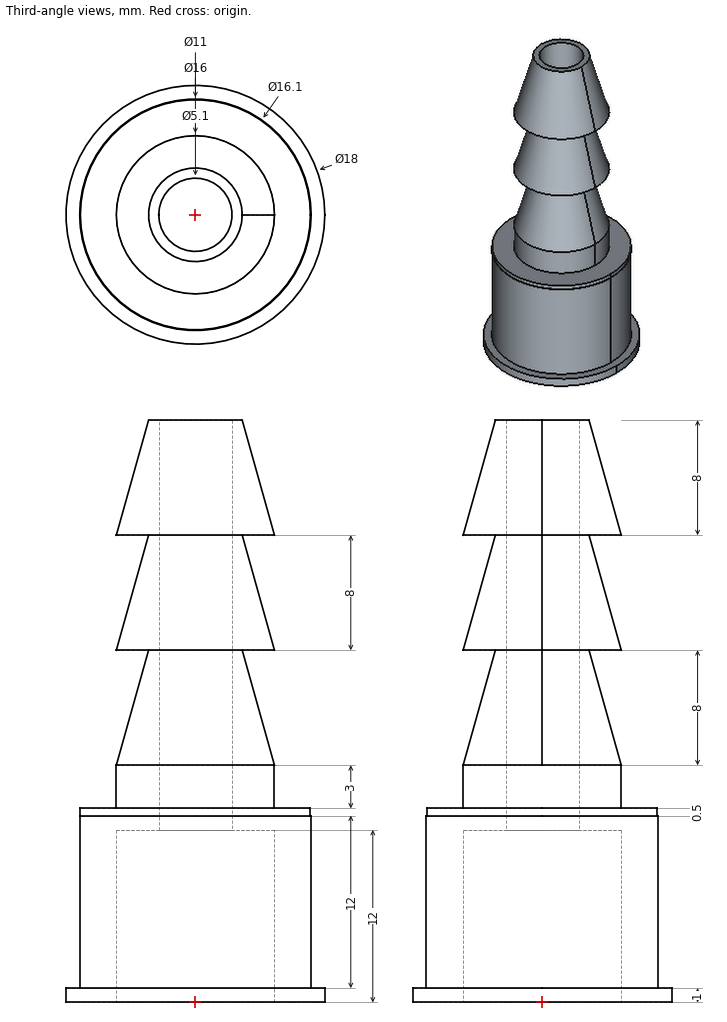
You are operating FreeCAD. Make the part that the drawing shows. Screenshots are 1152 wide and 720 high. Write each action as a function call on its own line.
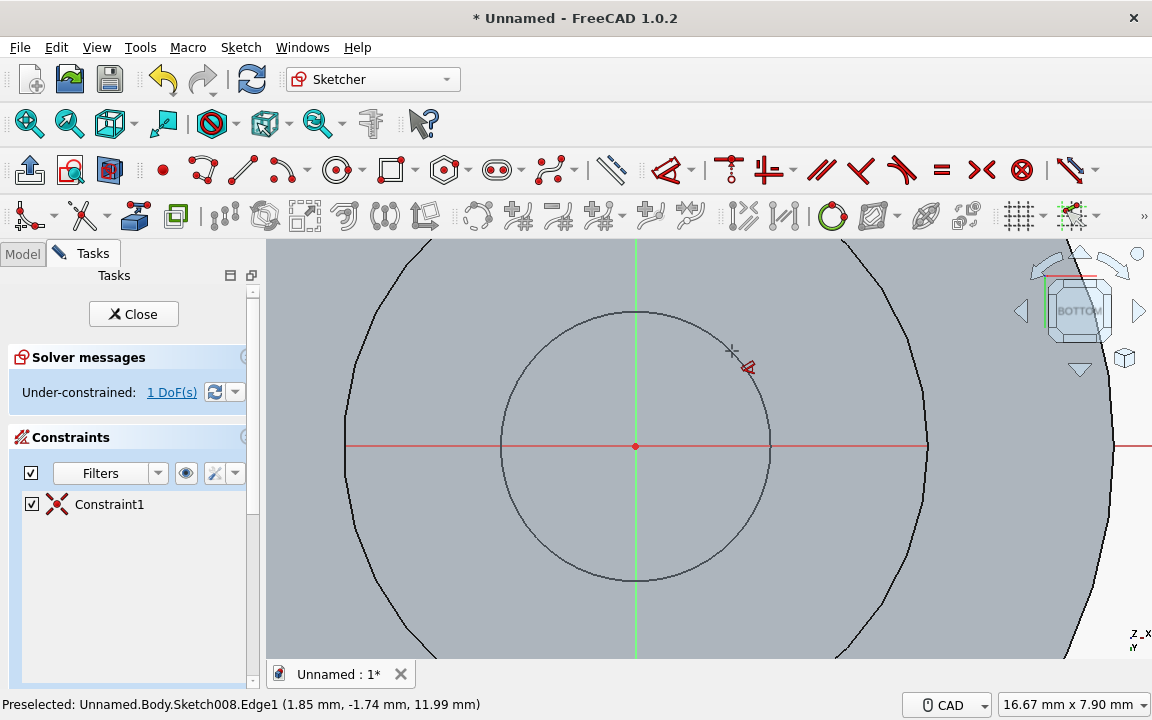
click(731, 351)
click(754, 328)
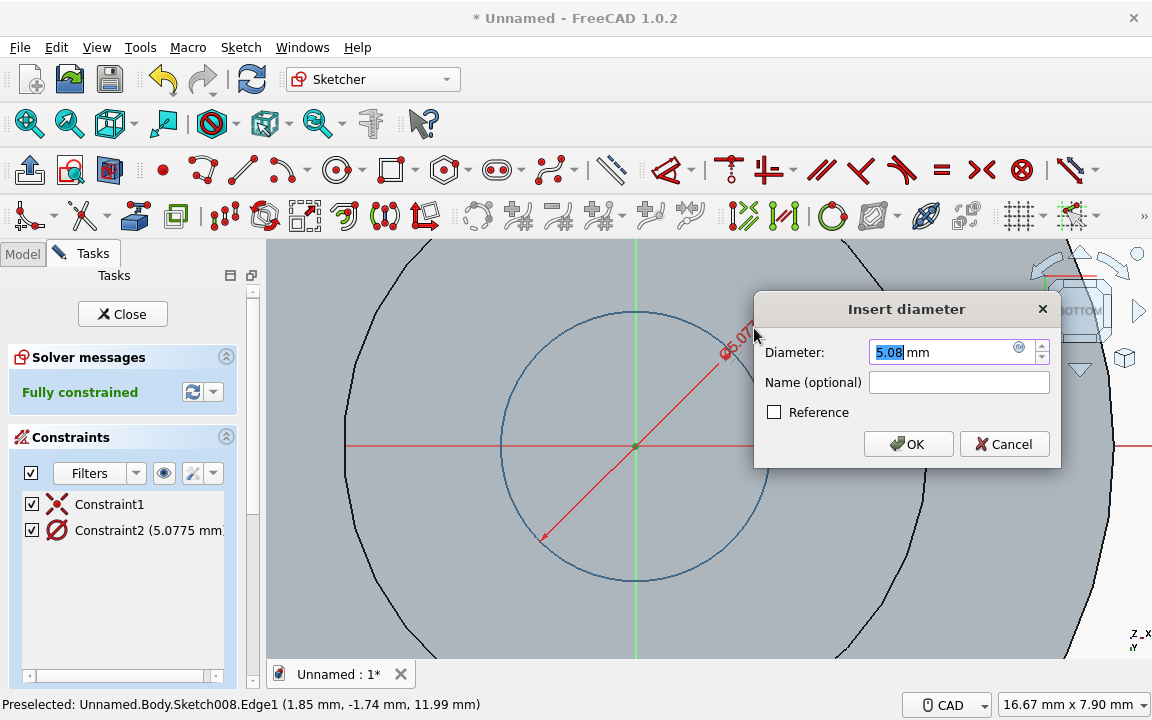
text(5.1)
key(Return)
key(Escape)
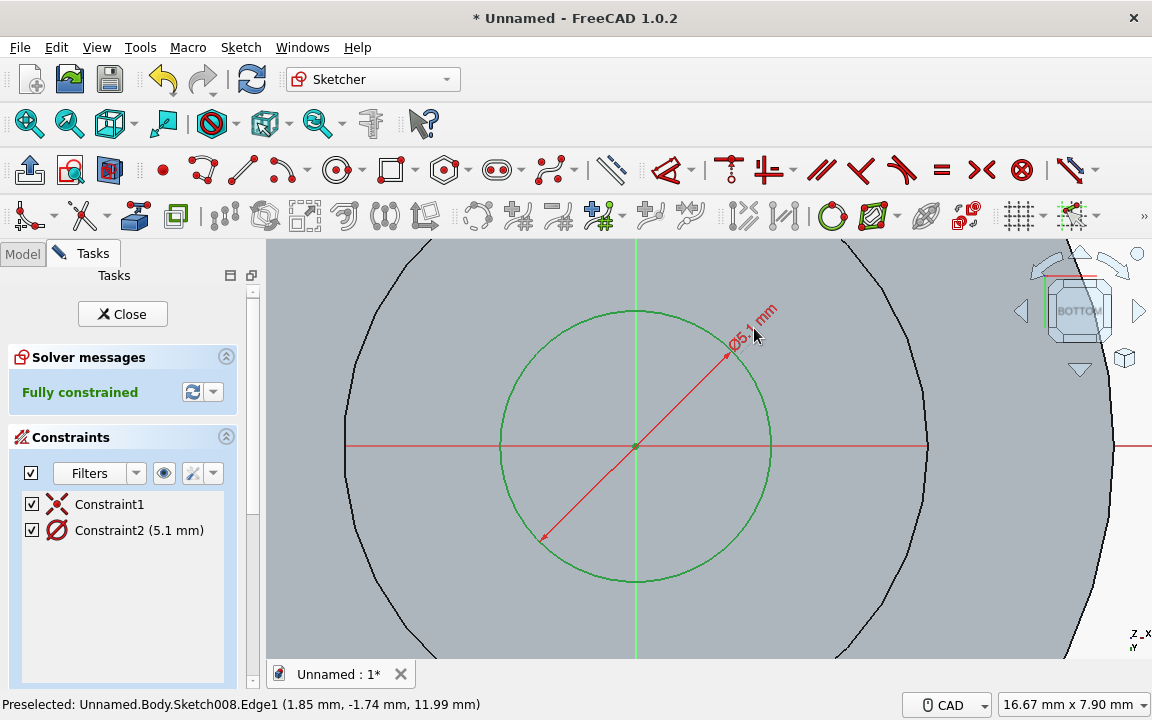
click(123, 314)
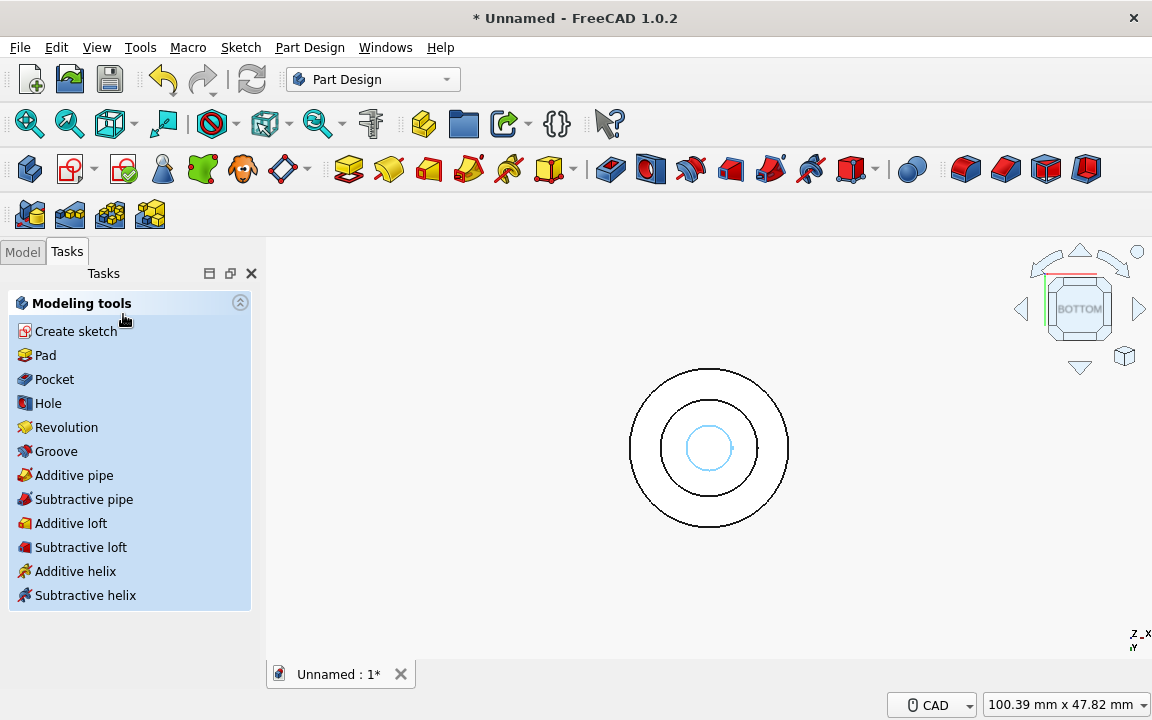
click(612, 170)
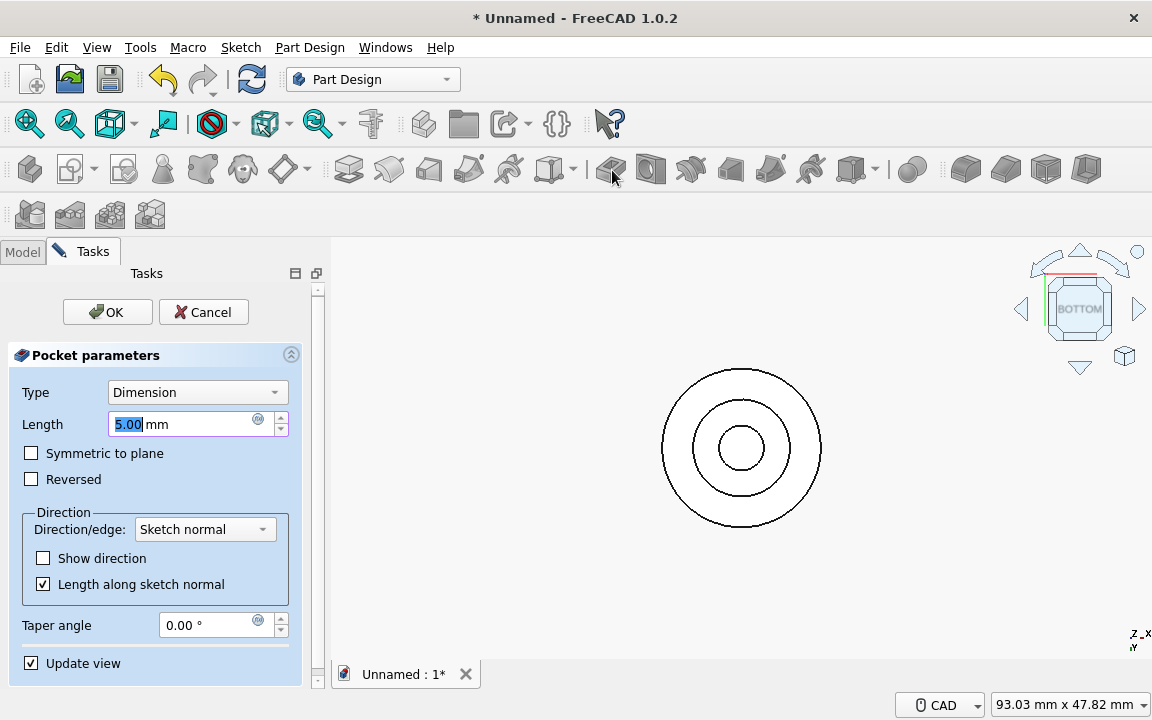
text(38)
key(Tab)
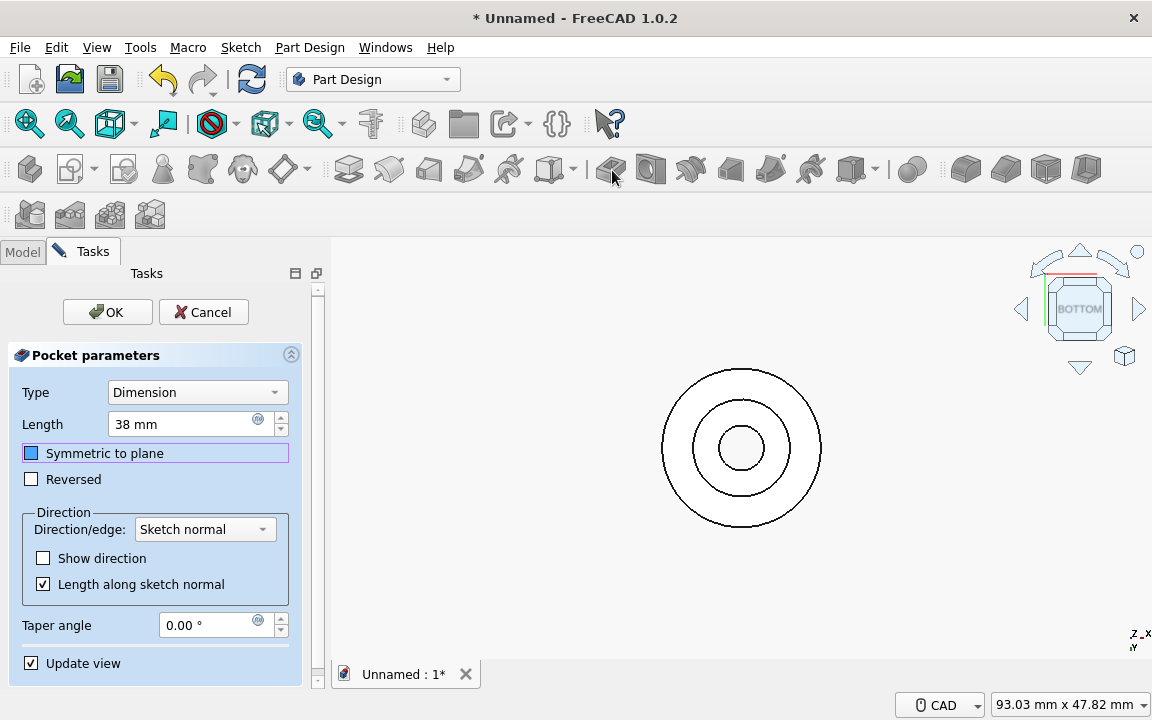
click(108, 312)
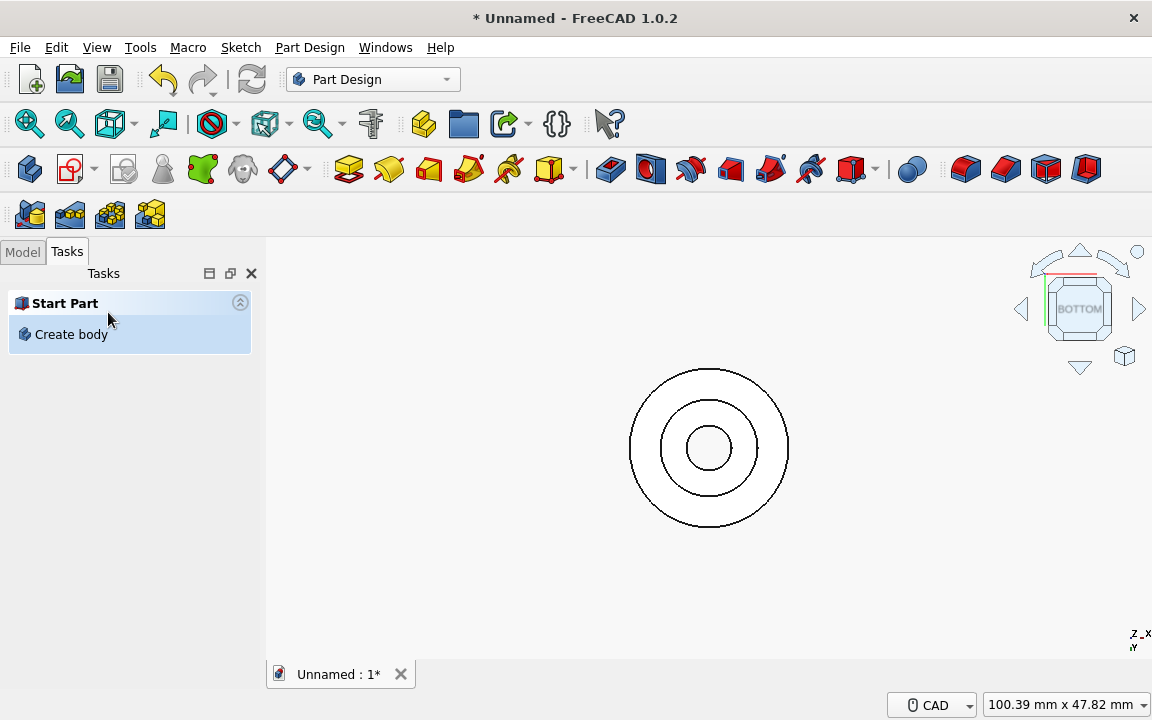
key(0)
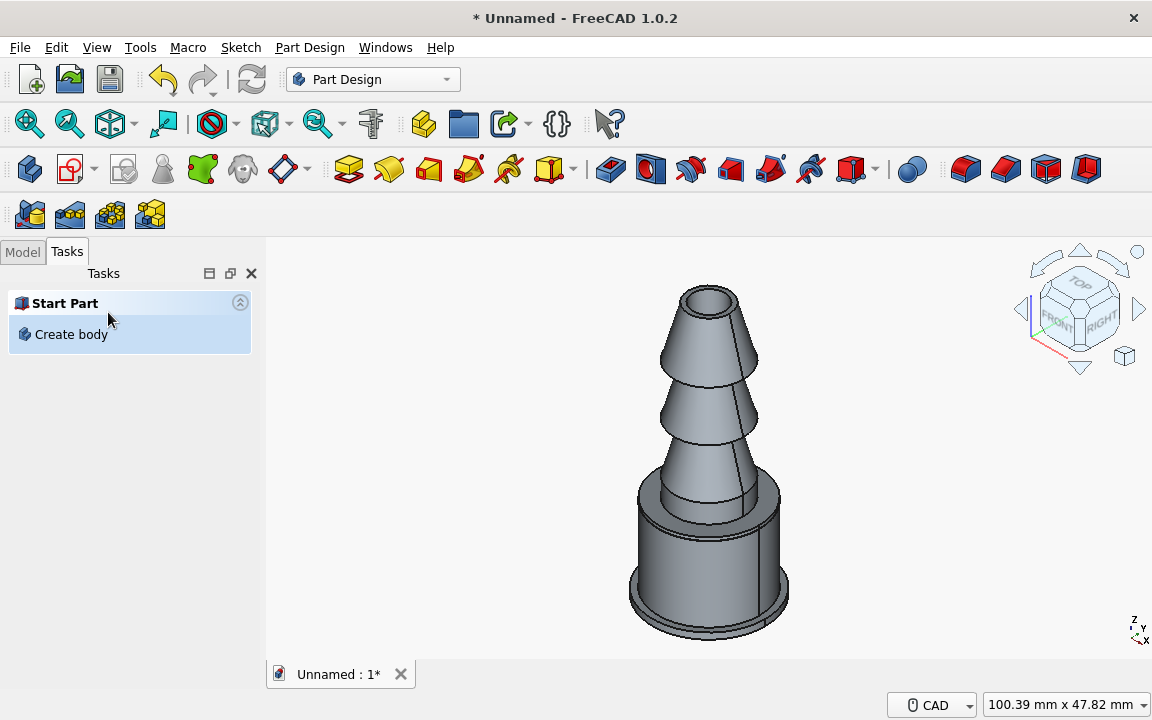
key(v)
key(f)